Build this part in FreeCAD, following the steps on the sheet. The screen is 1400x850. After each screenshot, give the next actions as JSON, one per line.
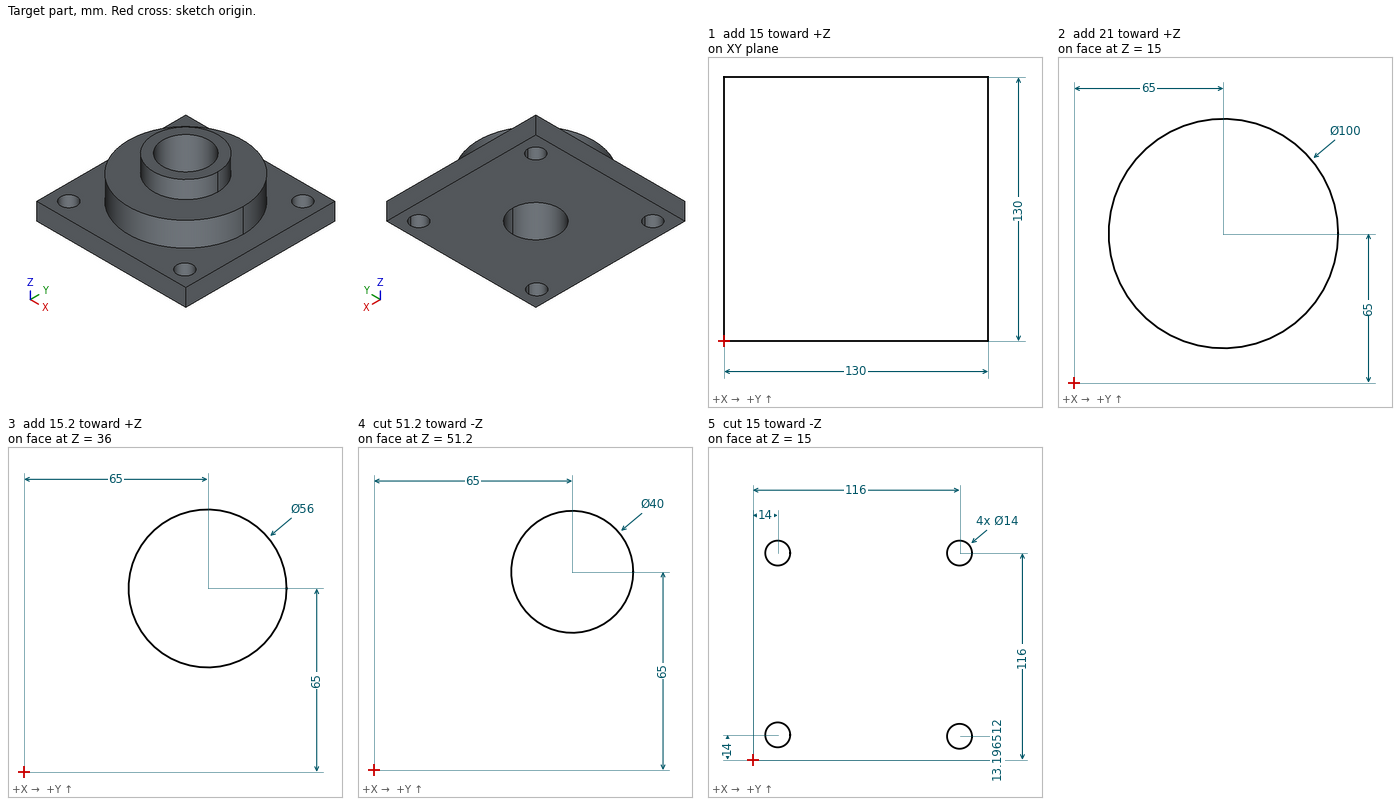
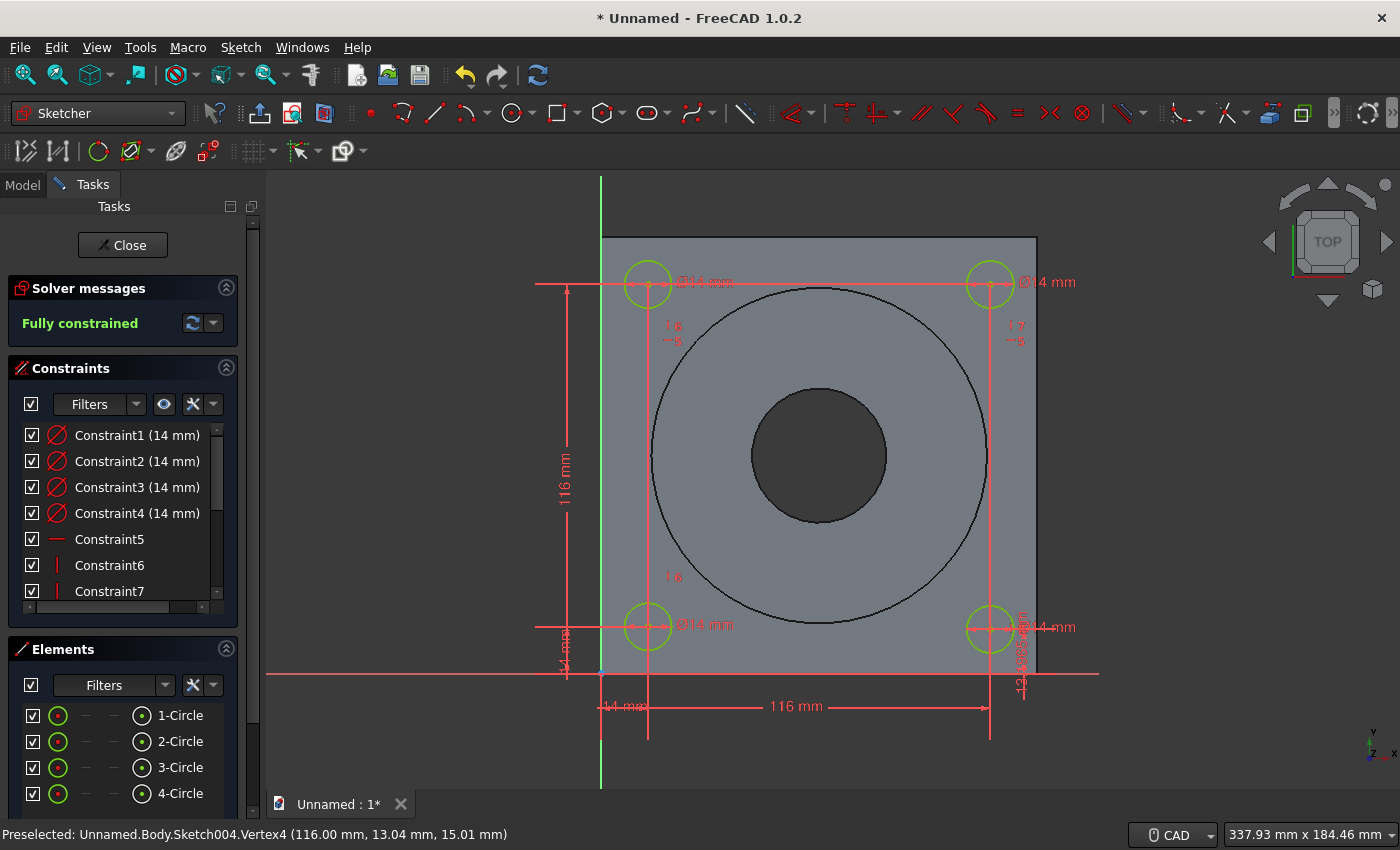
{"action": "left_click", "coordinate": [123, 245]}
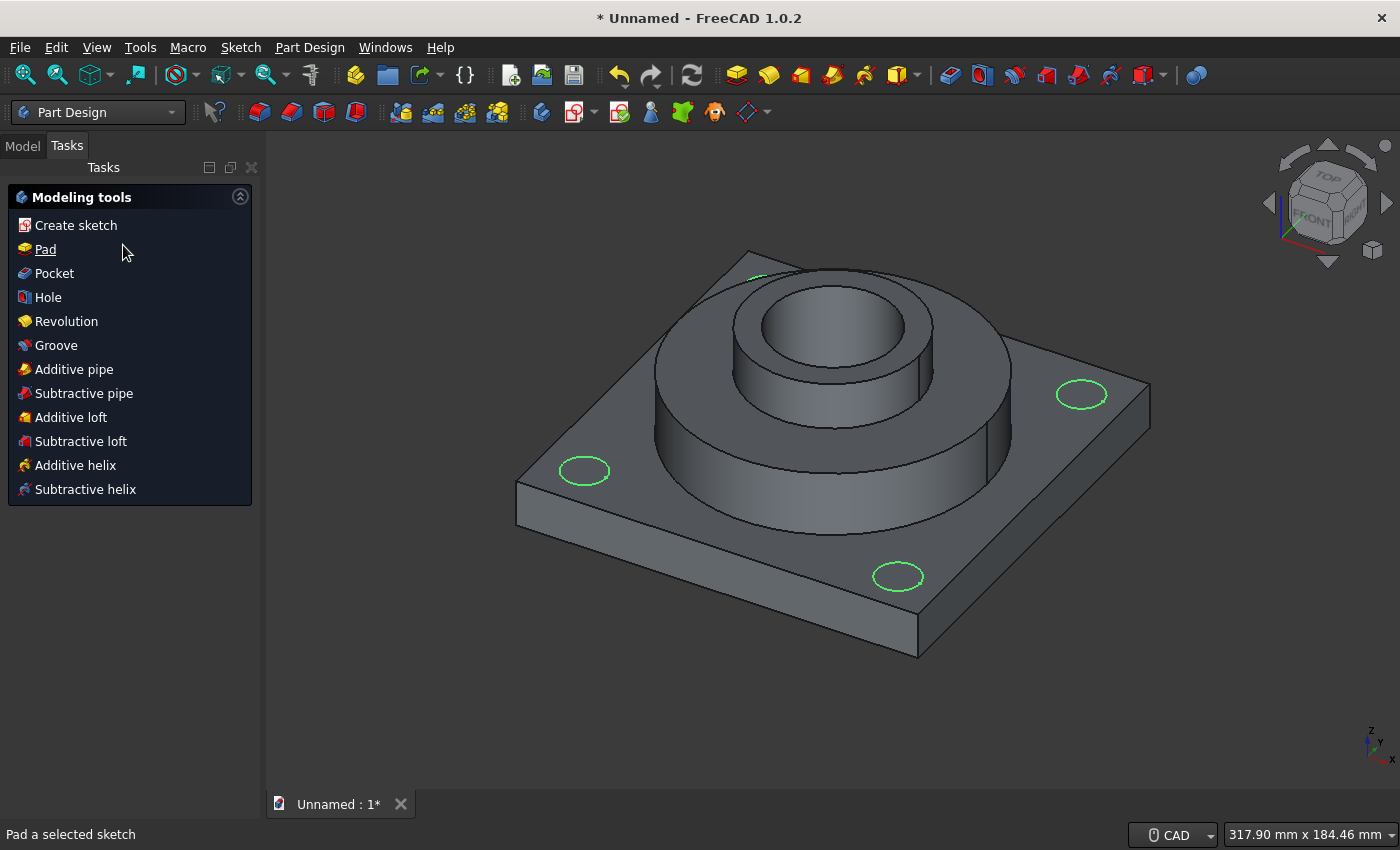
{"action": "left_click", "coordinate": [952, 76]}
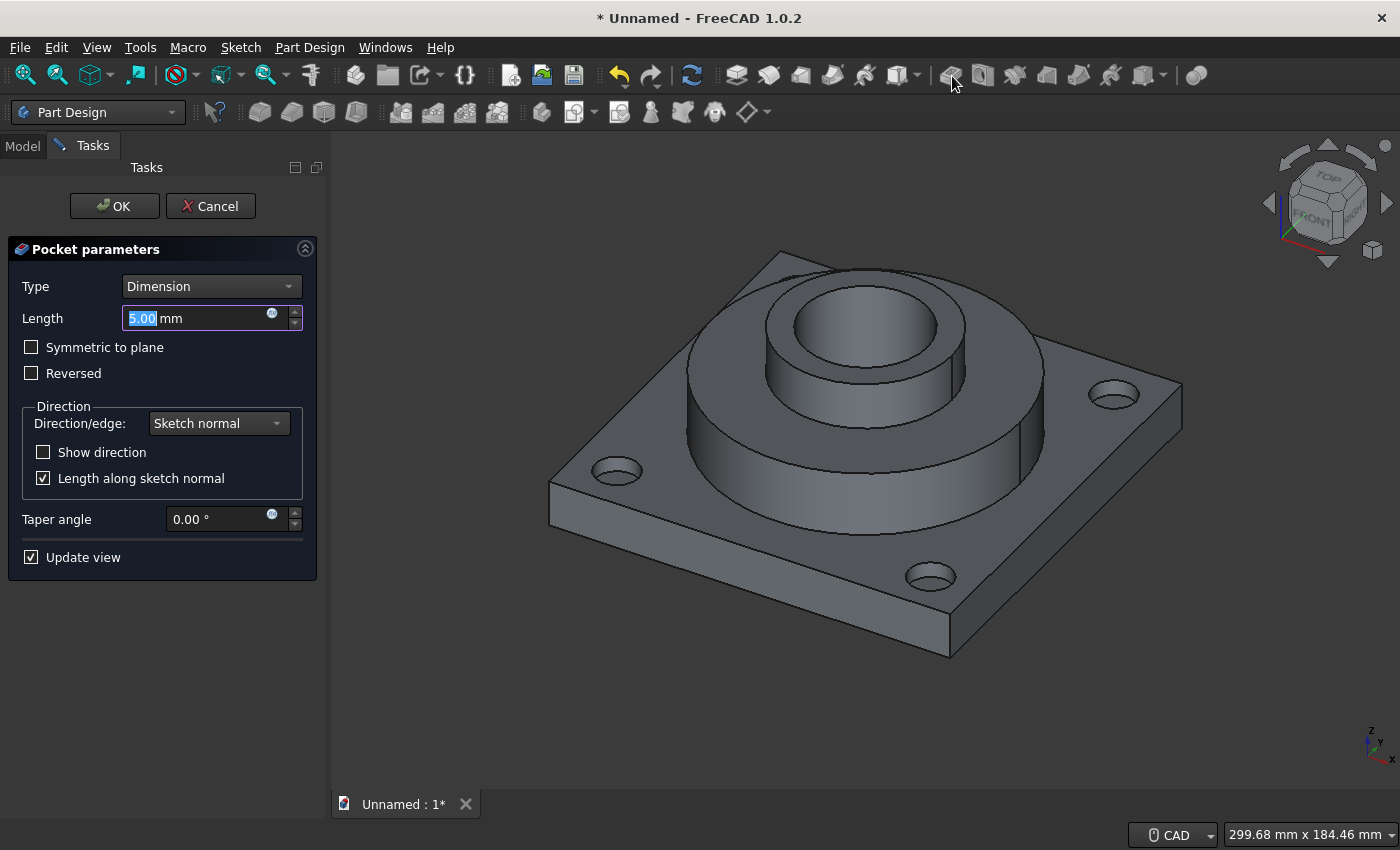
{"action": "type", "text": "15"}
{"action": "key", "text": "Tab"}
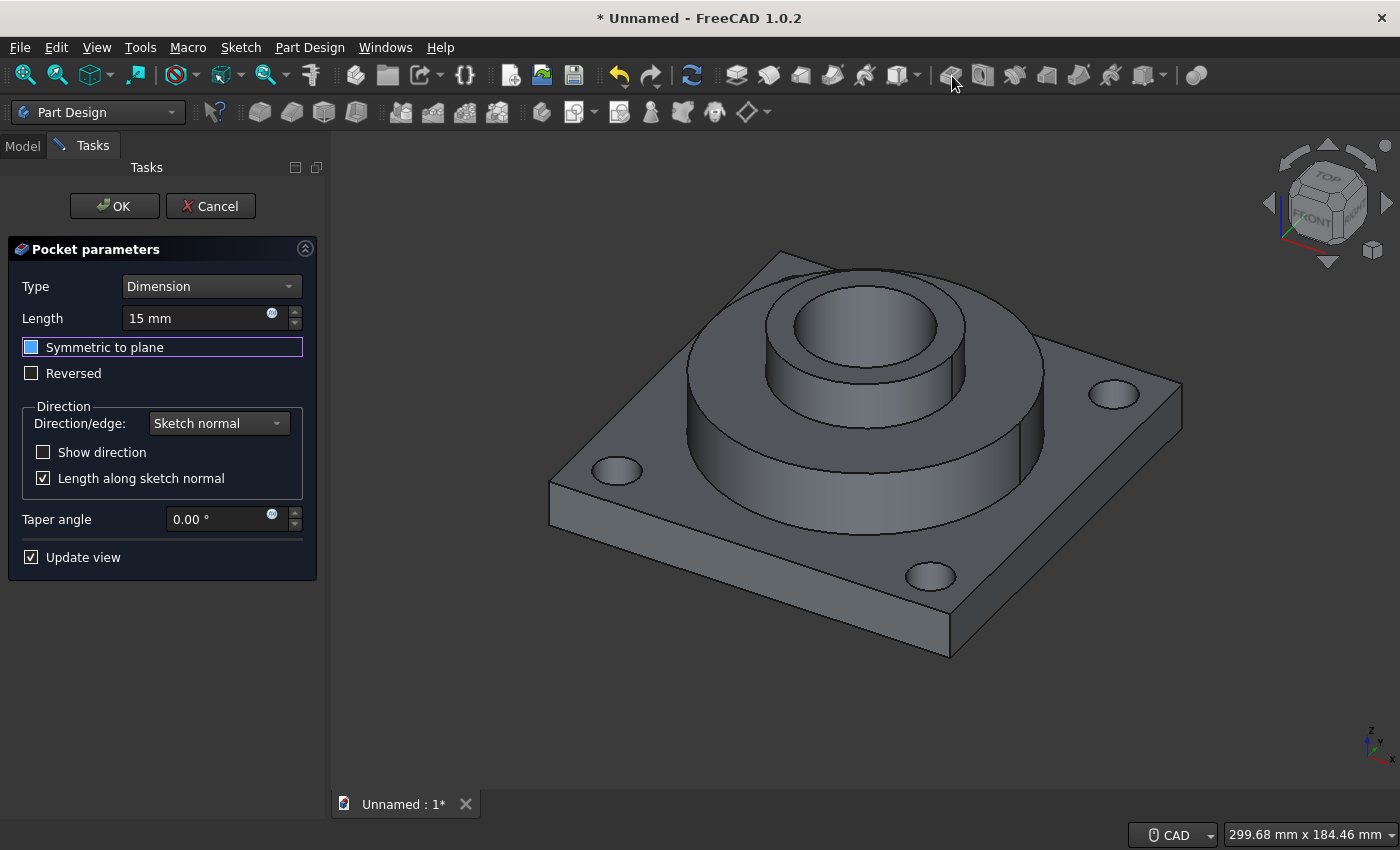
{"action": "left_click", "coordinate": [115, 206]}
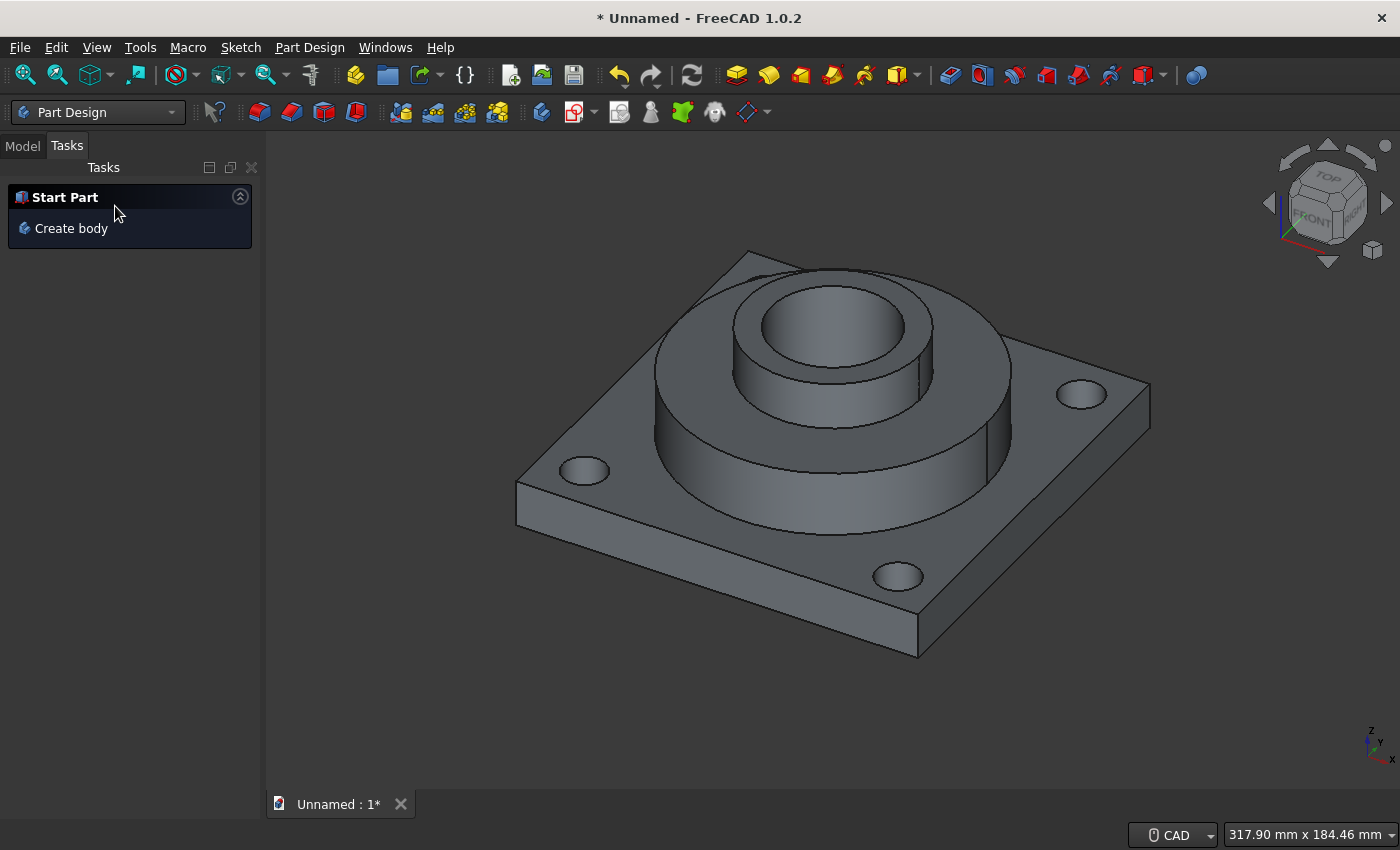
{"action": "key", "text": "0"}